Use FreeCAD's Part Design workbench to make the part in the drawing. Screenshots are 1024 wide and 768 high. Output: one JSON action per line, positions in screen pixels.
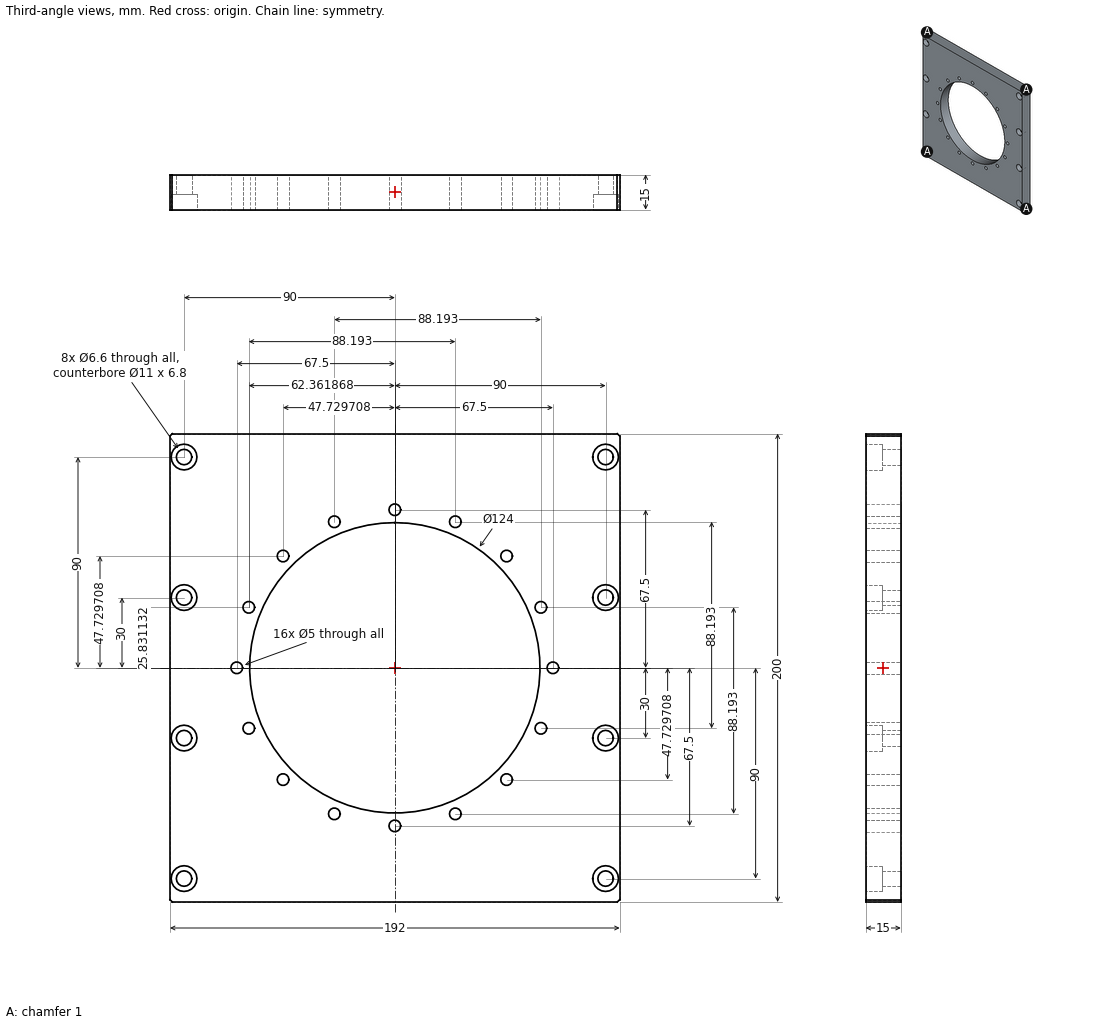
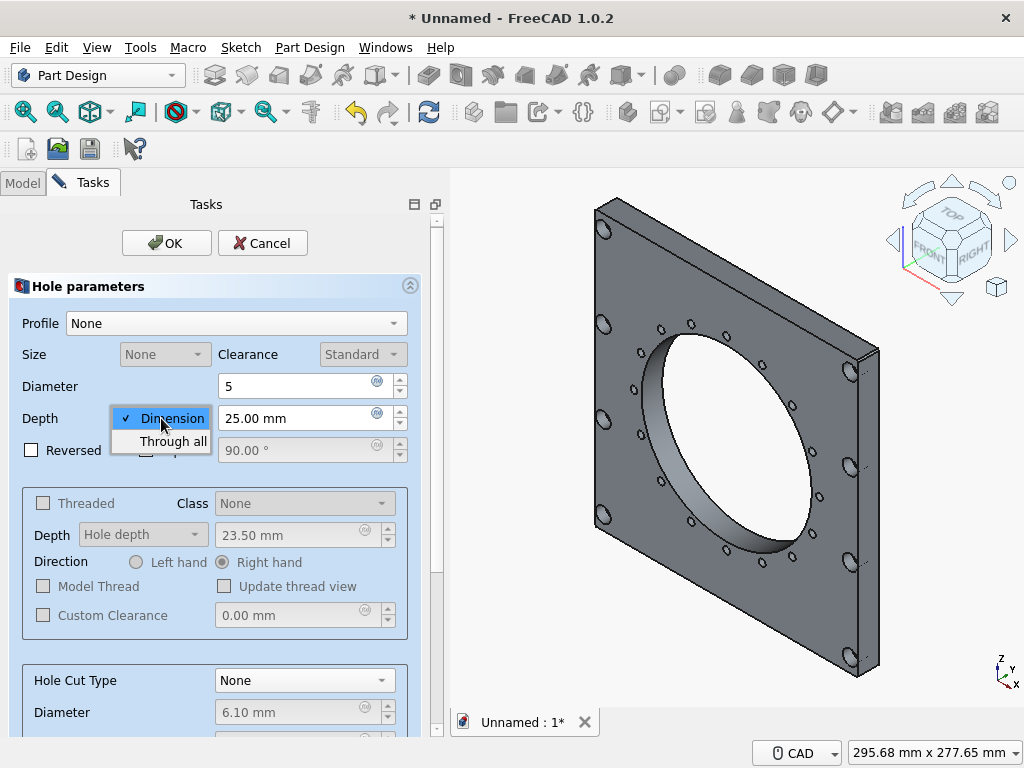
{"action": "left_click", "coordinate": [160, 442]}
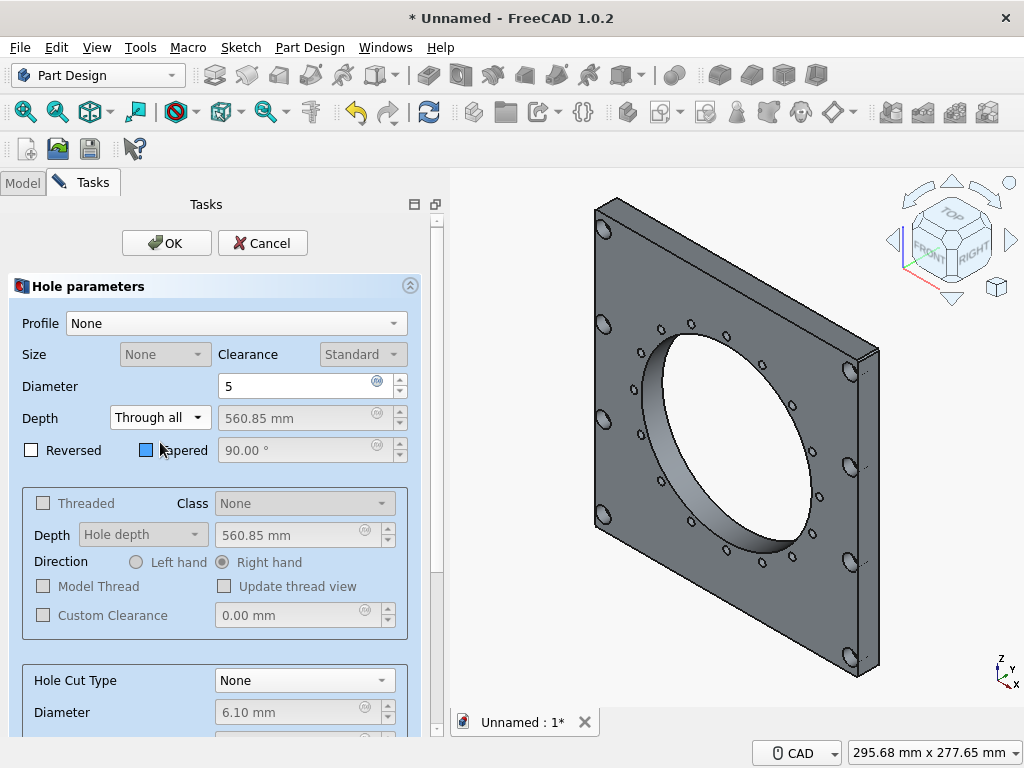
{"action": "left_click", "coordinate": [167, 243]}